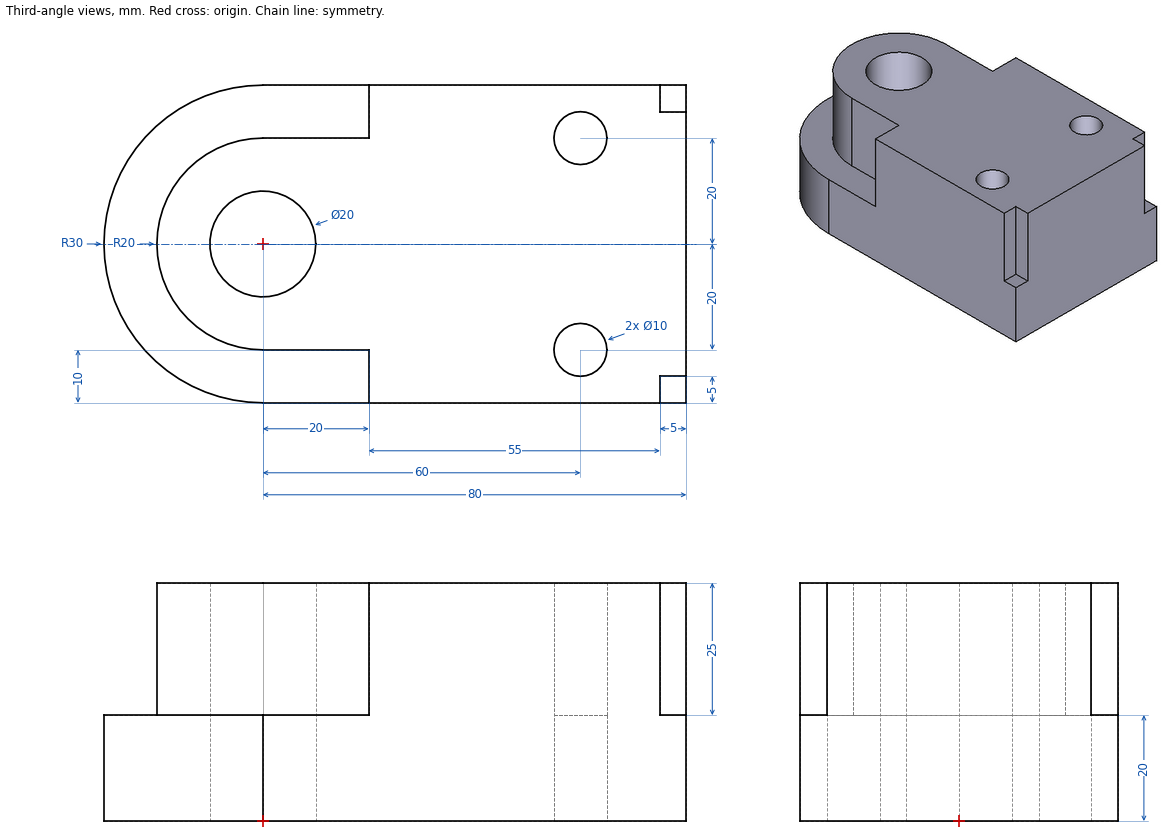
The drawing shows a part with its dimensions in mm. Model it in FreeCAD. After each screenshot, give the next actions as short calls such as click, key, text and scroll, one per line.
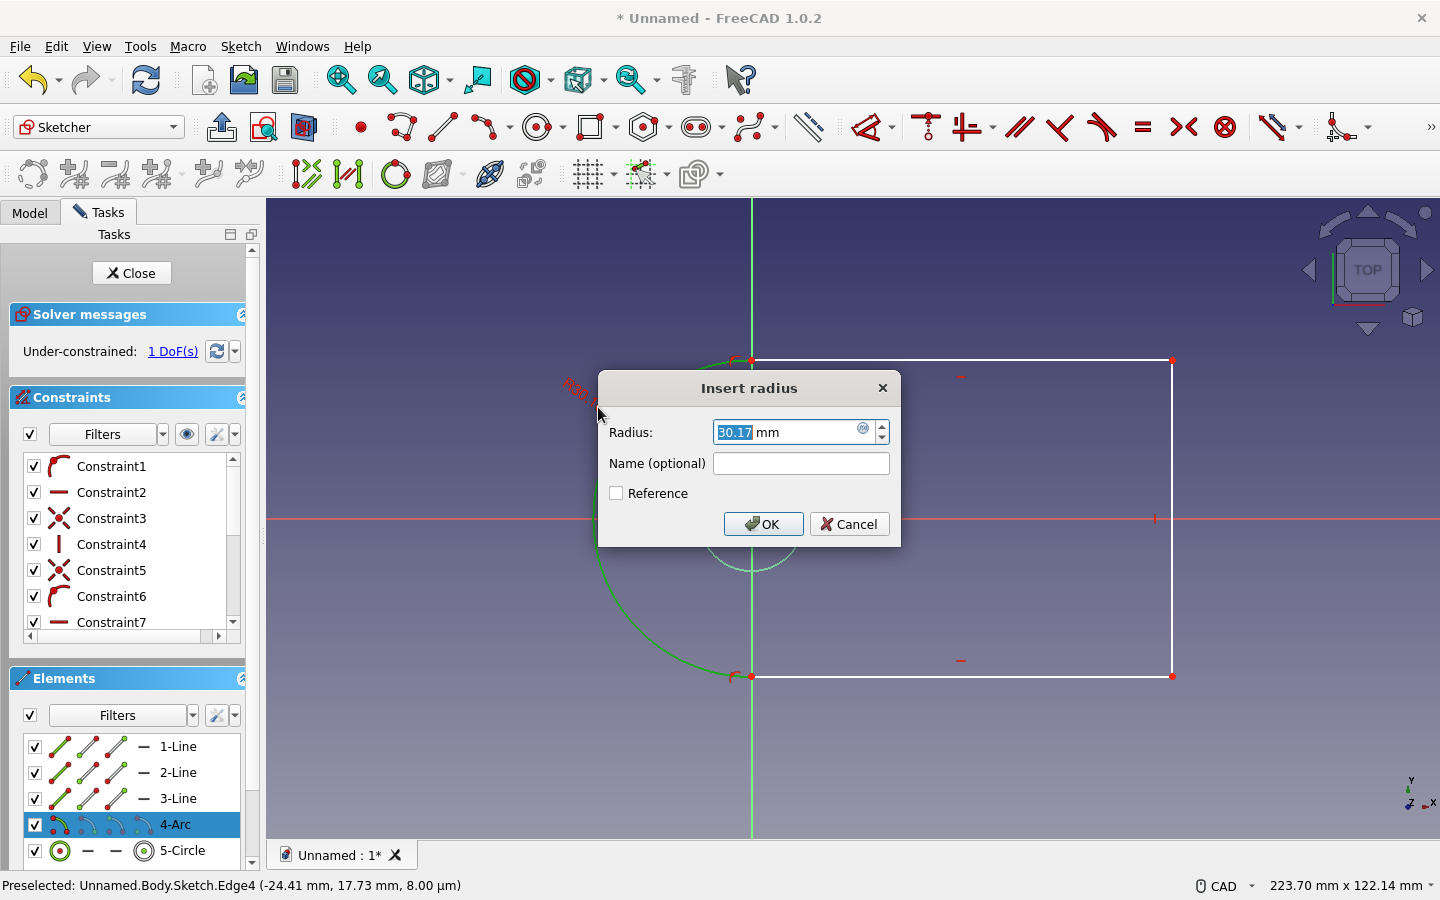
text(30)
key(Return)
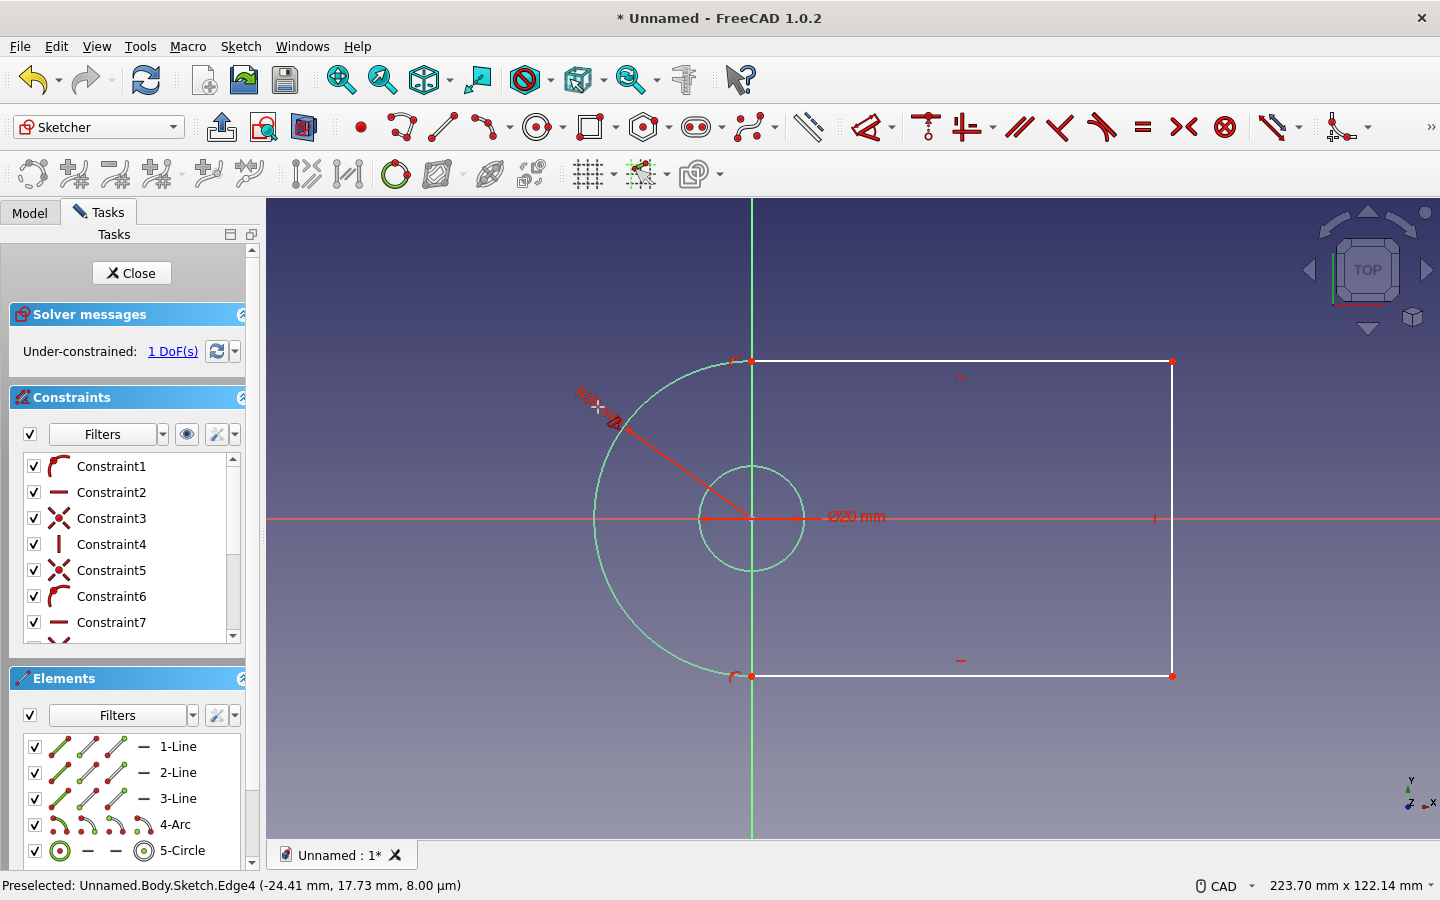
click(878, 676)
click(962, 710)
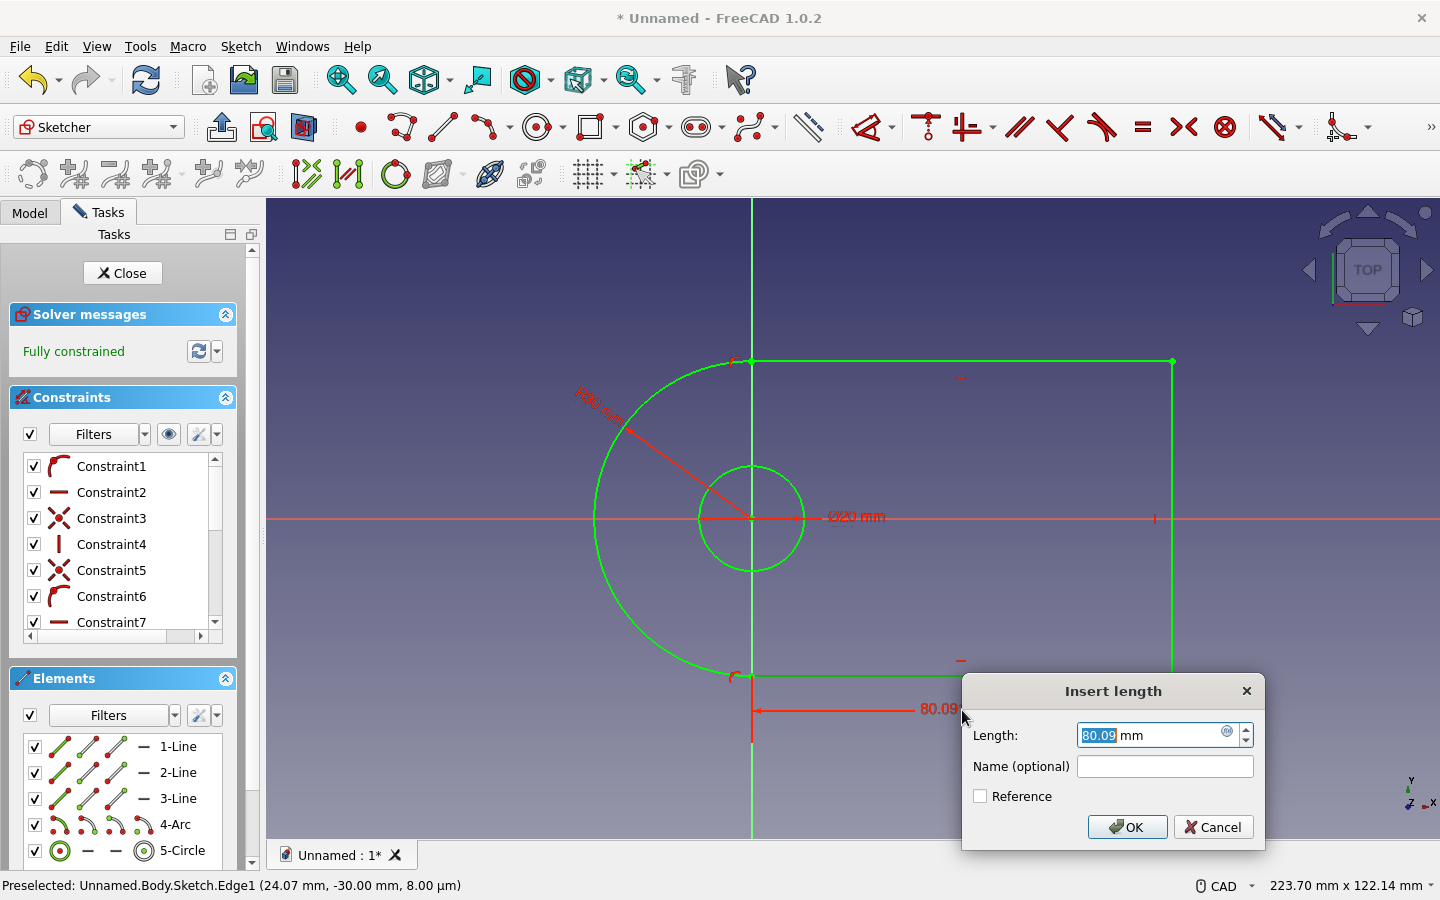
text(80)
key(Return)
key(Escape)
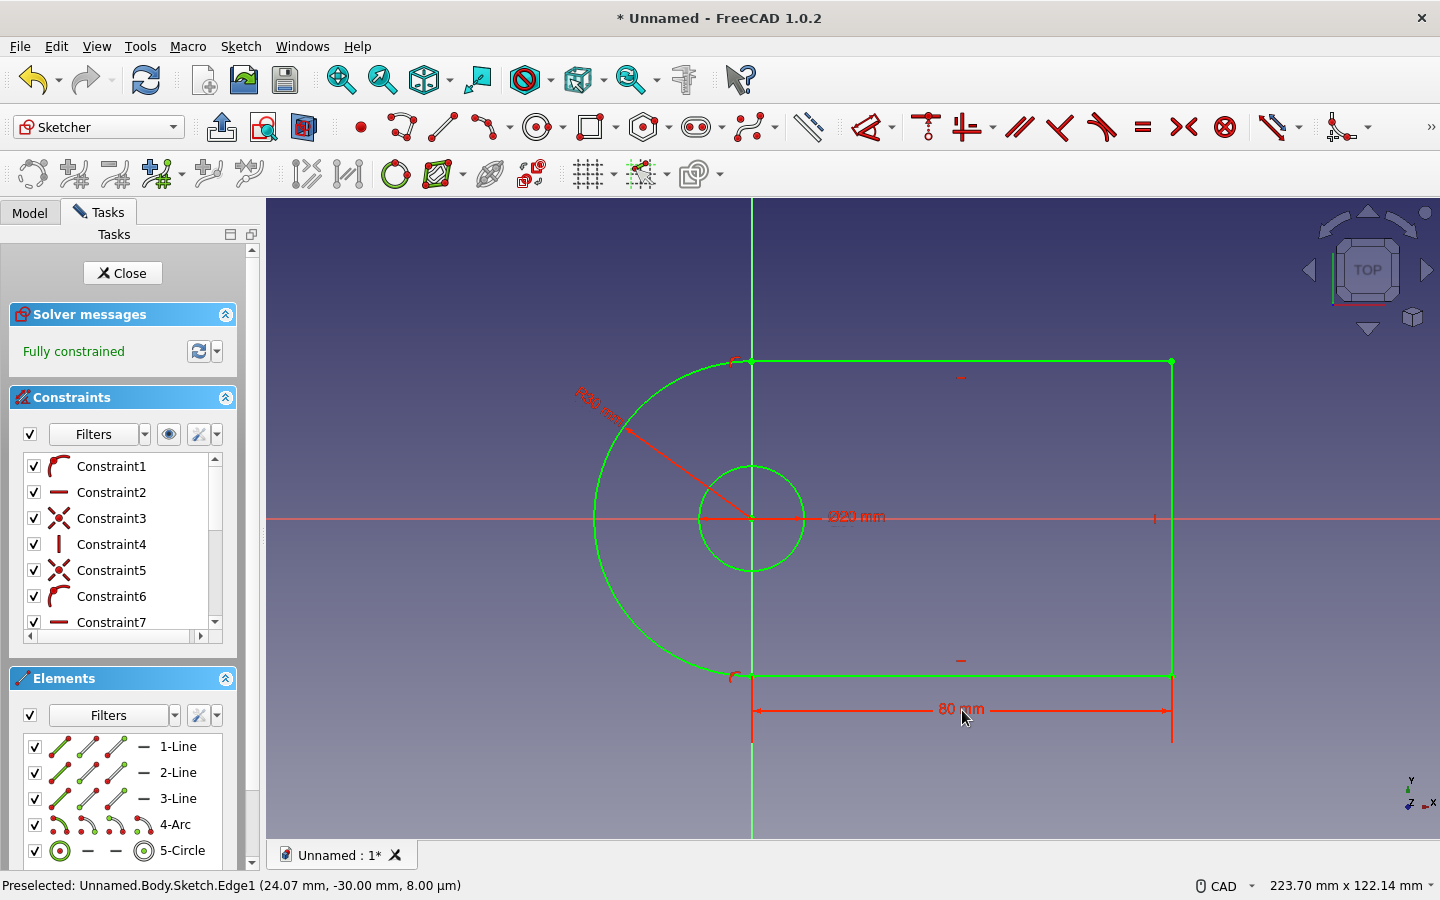
click(123, 273)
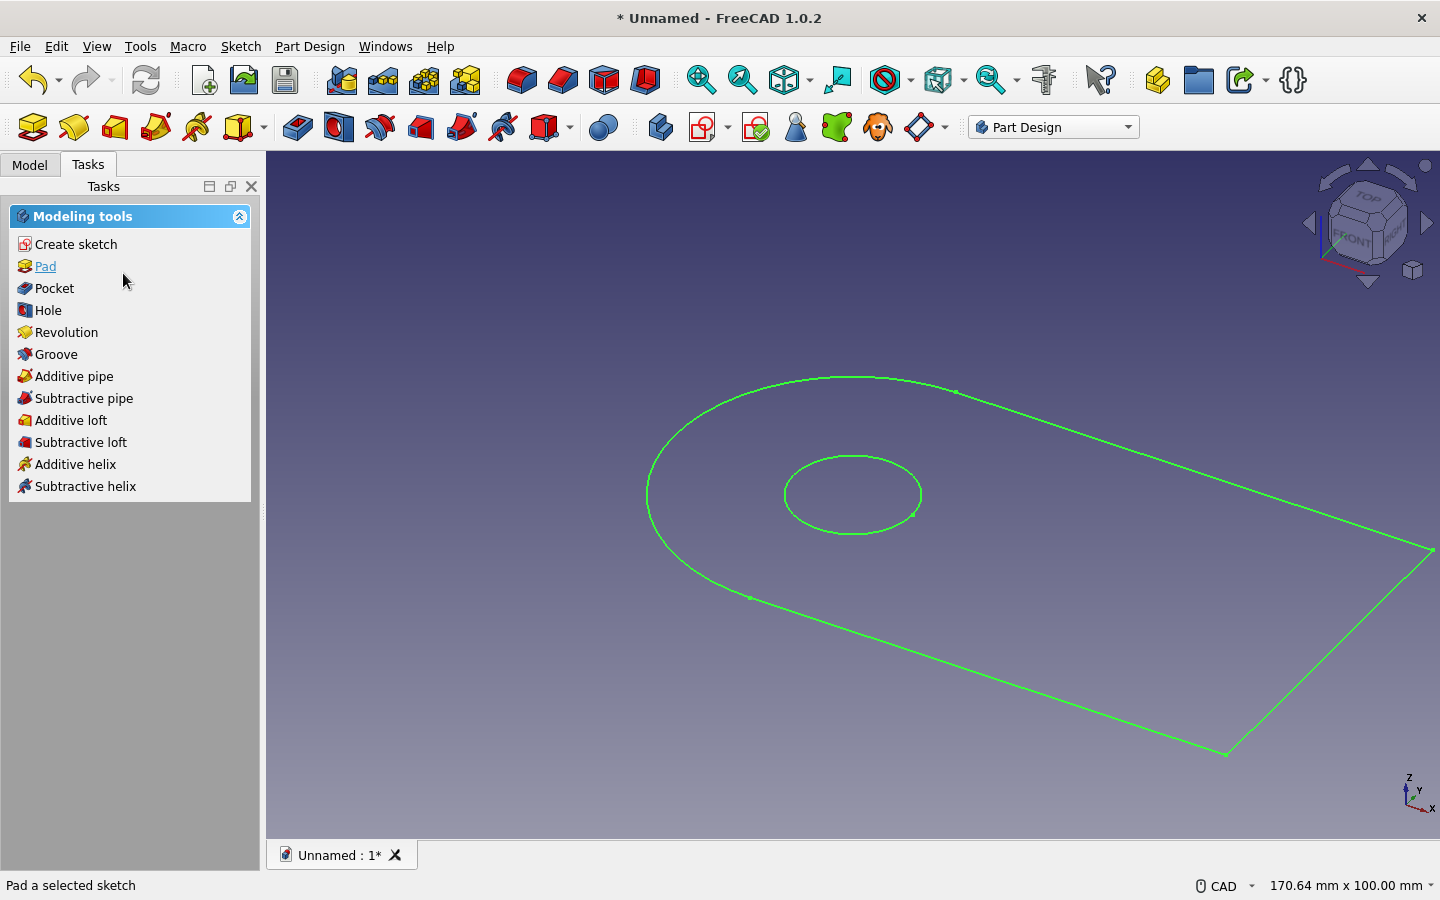
click(33, 128)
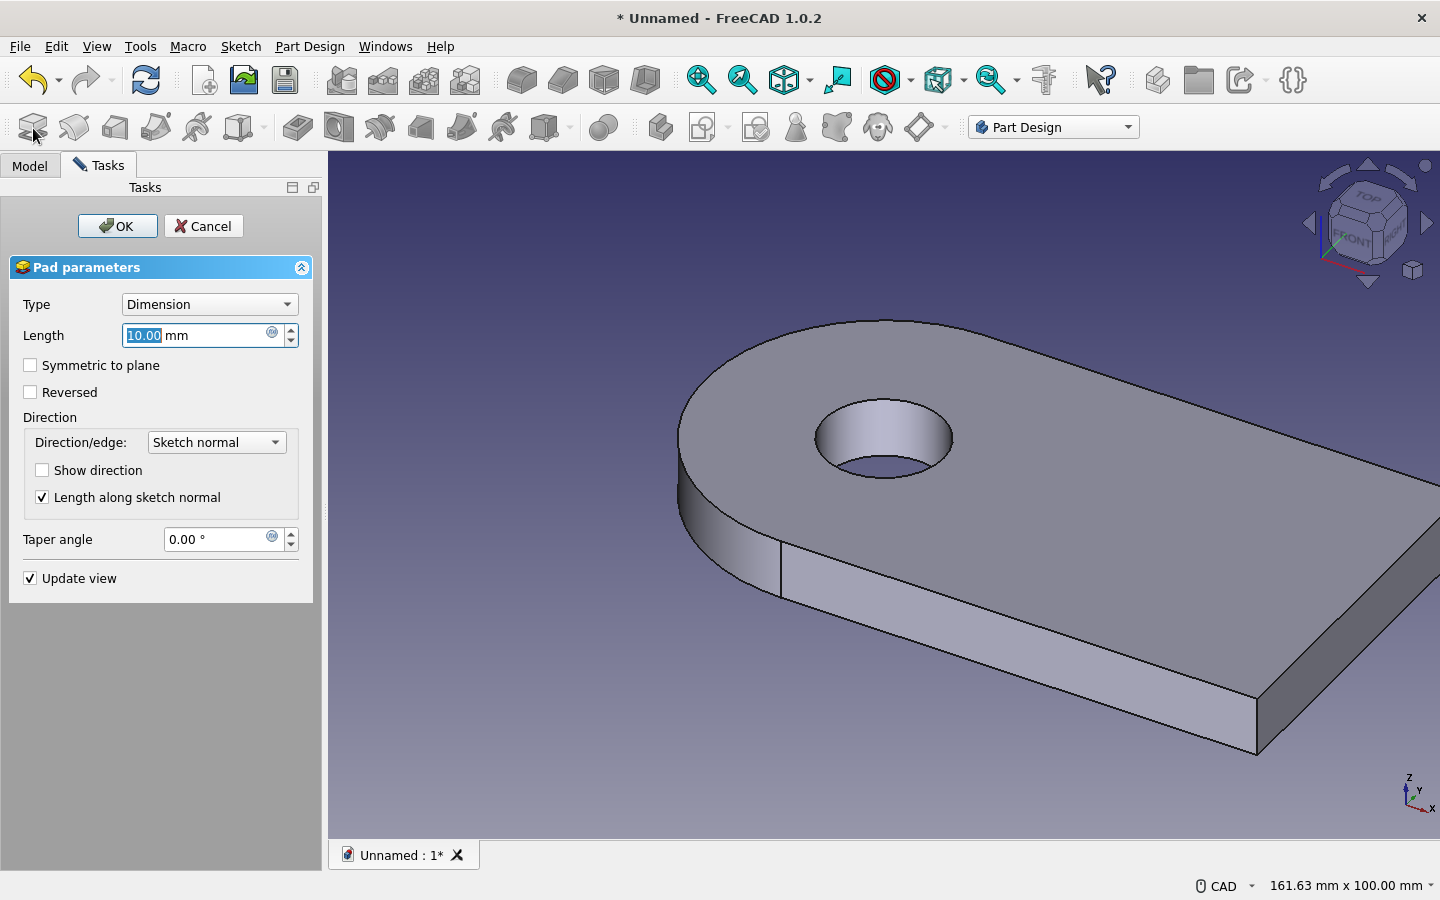
text(20)
key(Tab)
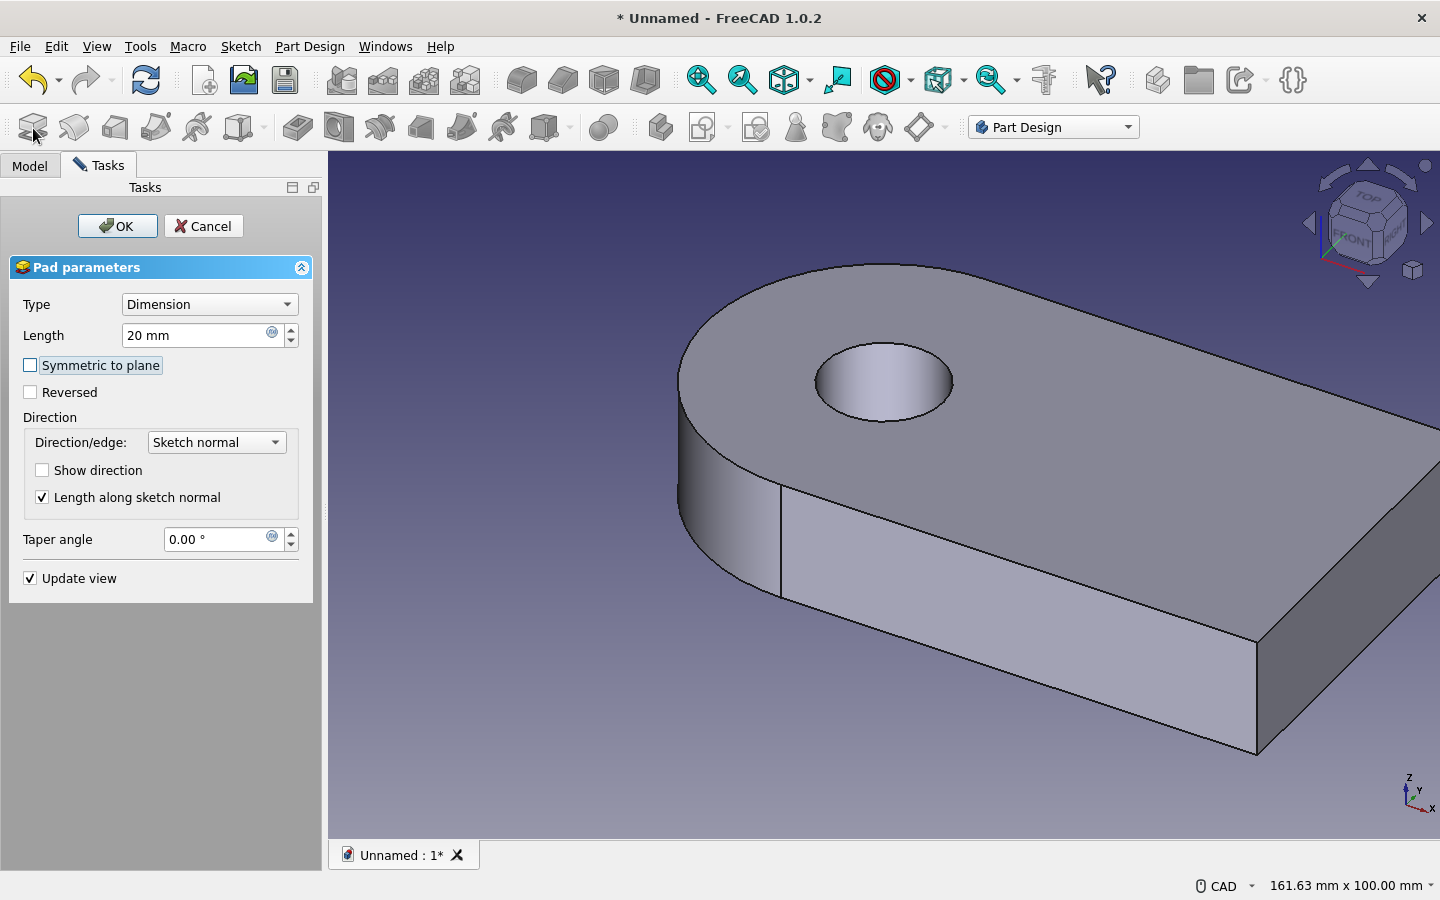
click(118, 226)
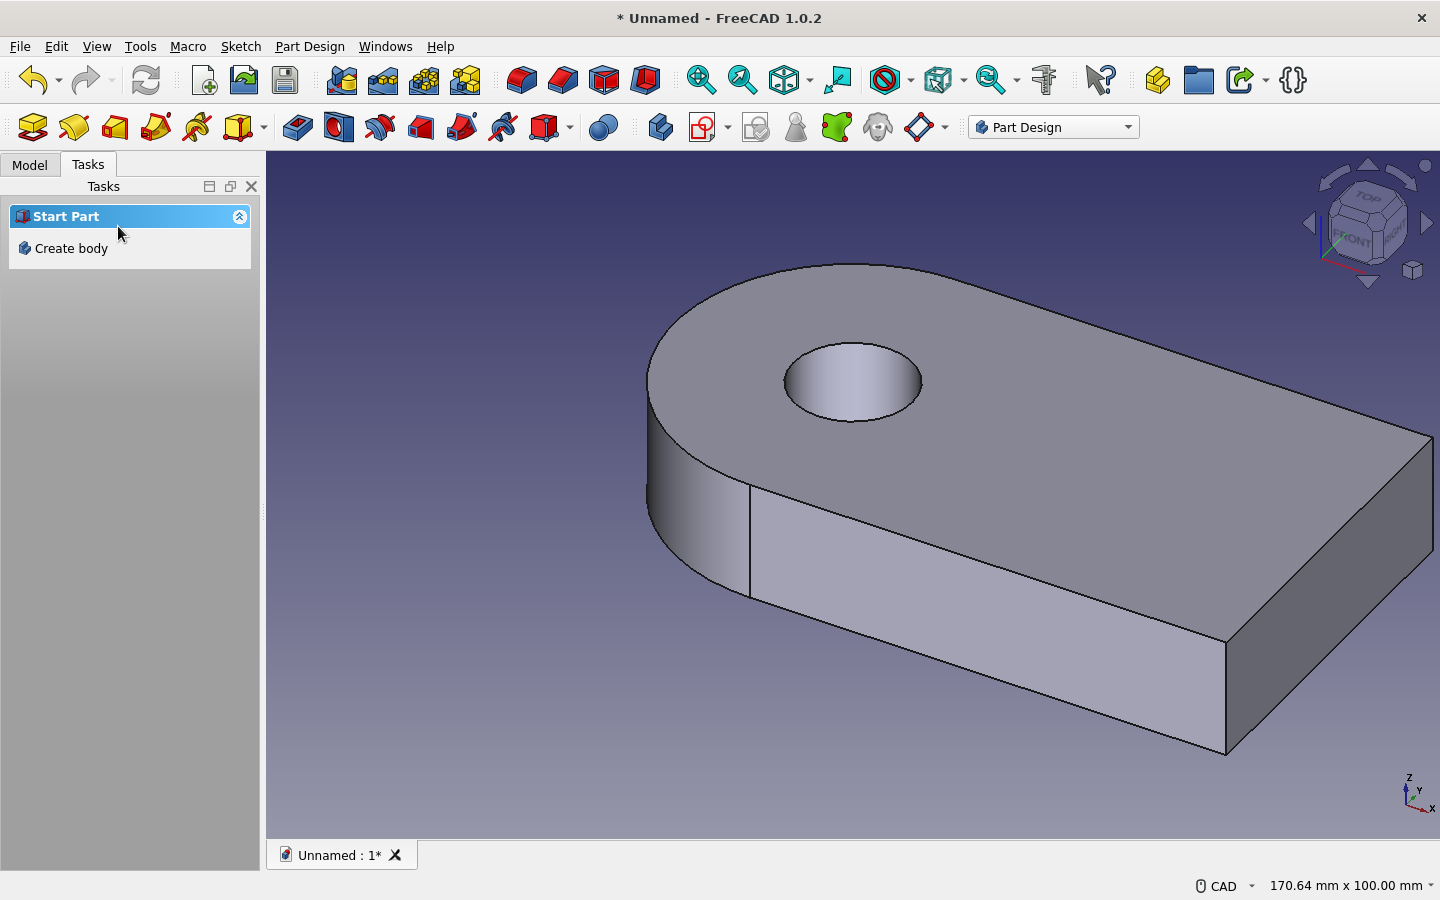
click(1096, 462)